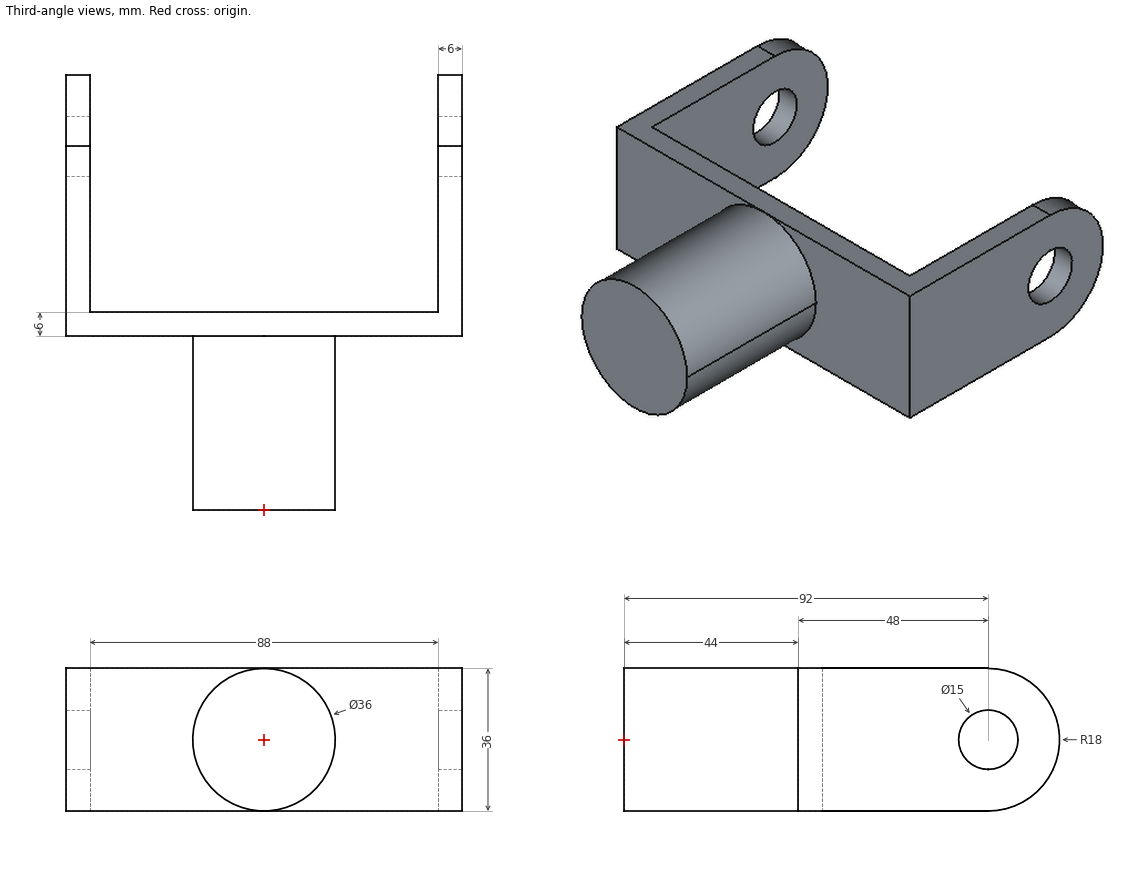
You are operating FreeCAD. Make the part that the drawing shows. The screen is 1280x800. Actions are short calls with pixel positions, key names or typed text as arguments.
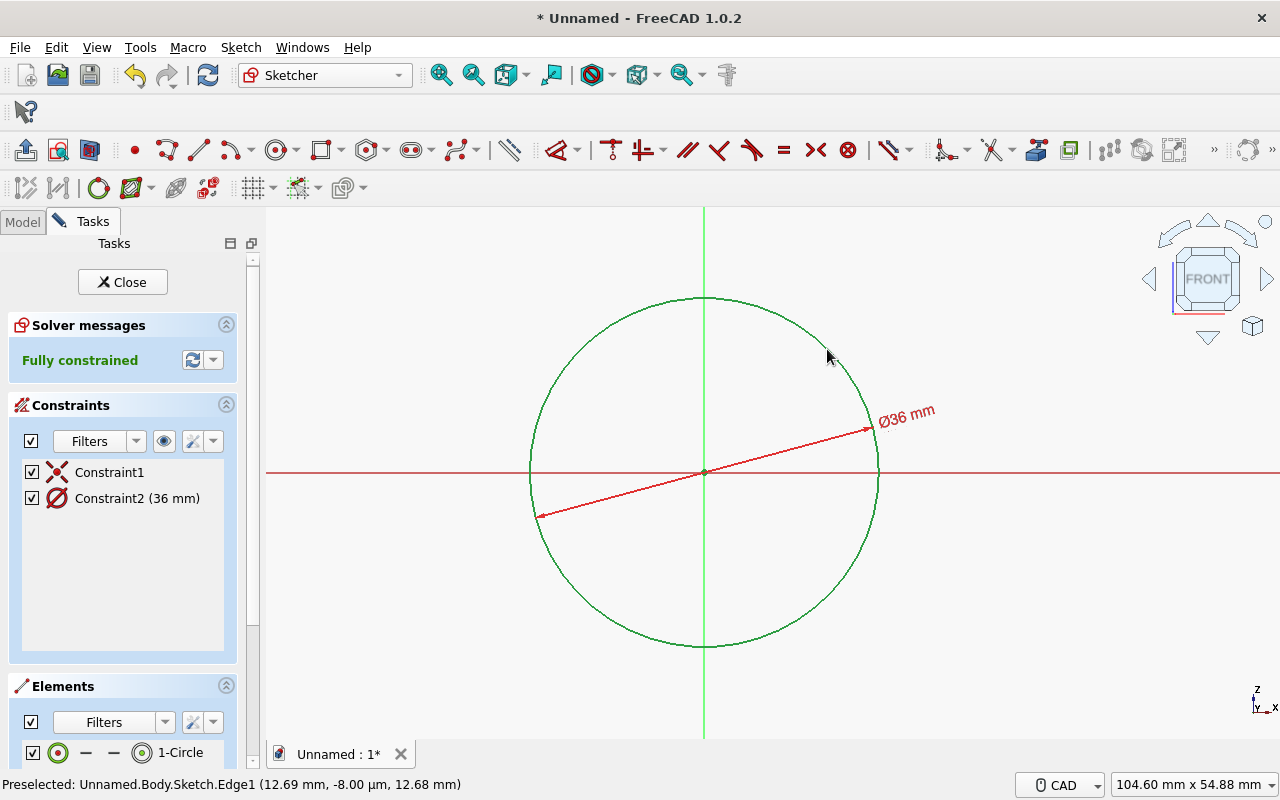
click(123, 282)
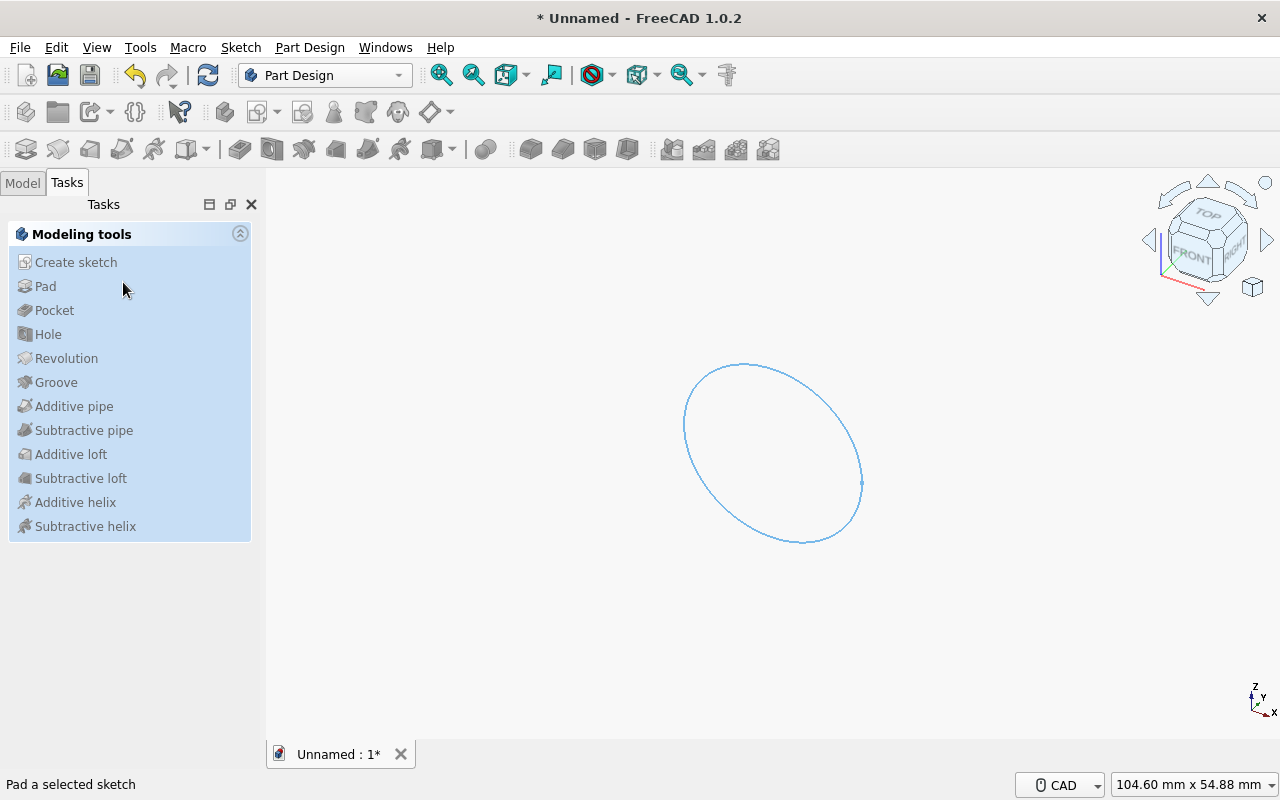
click(26, 150)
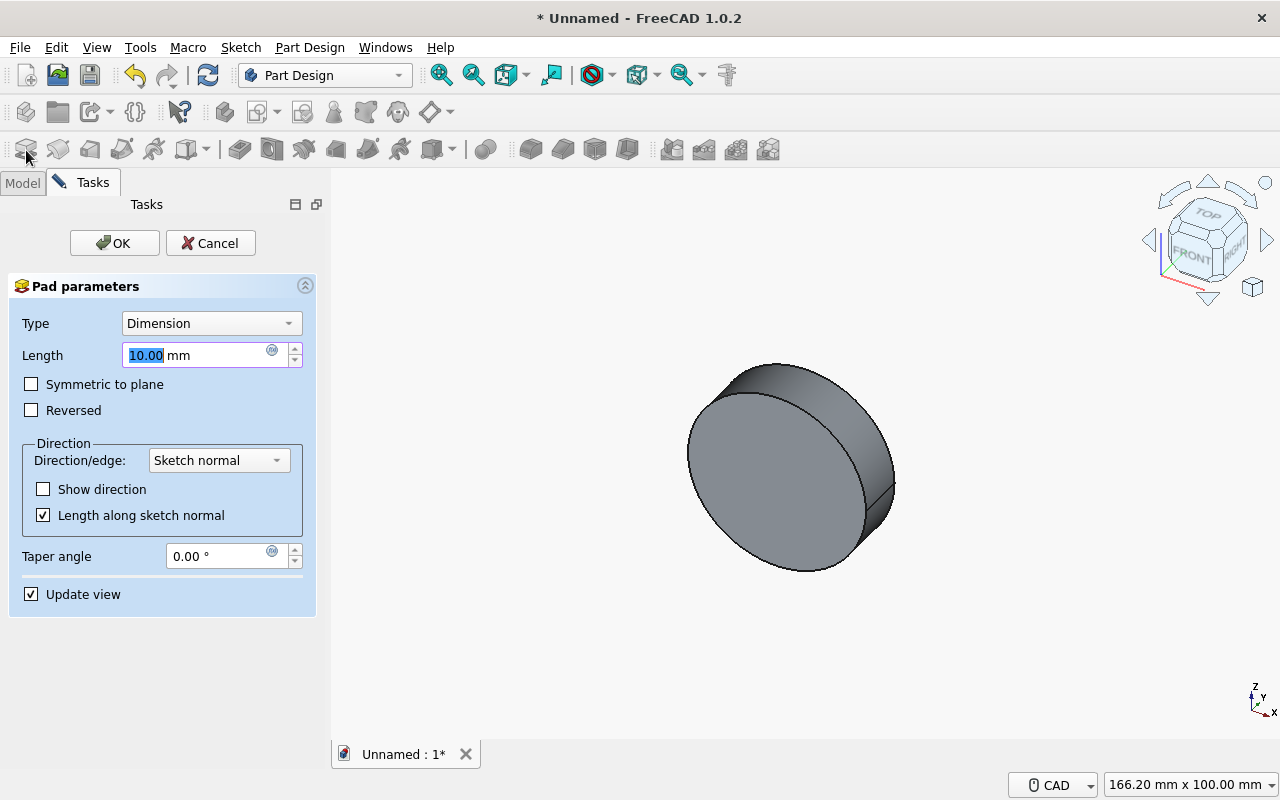
text(44)
key(Tab)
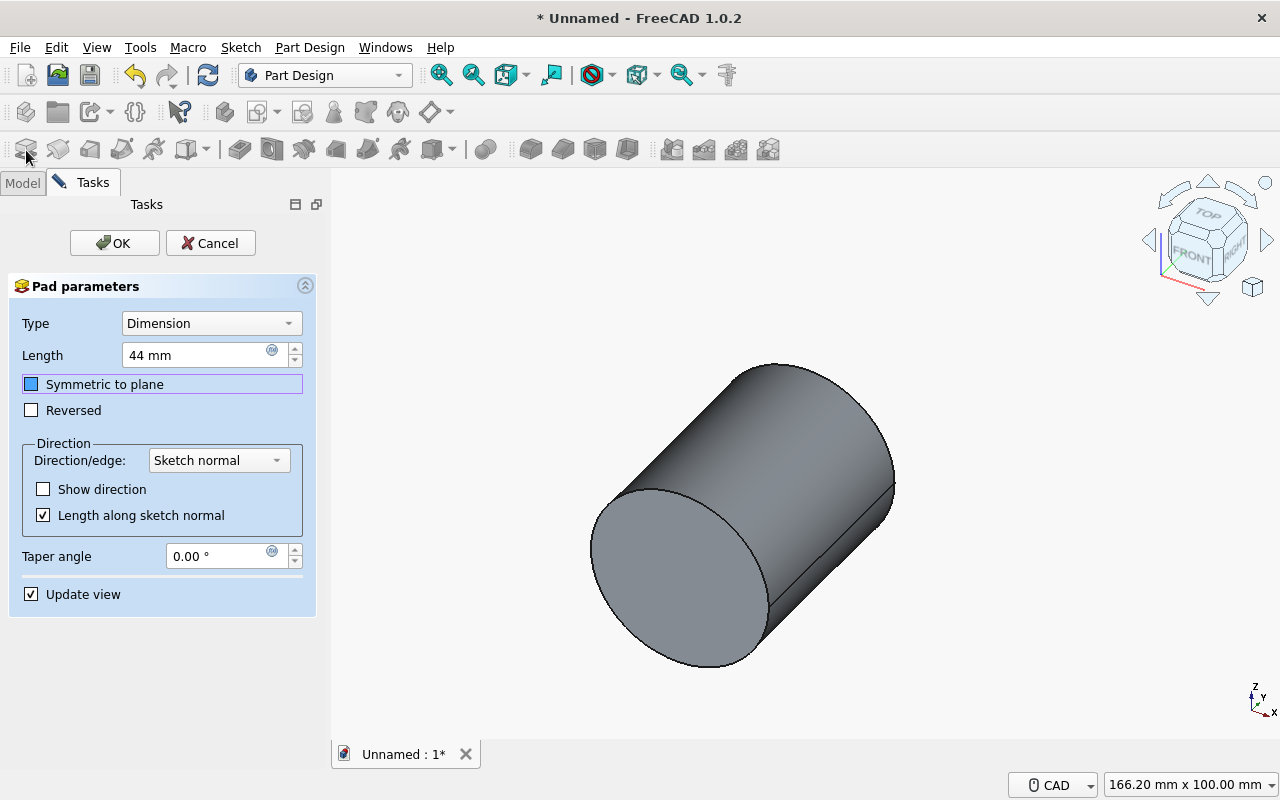
click(30, 410)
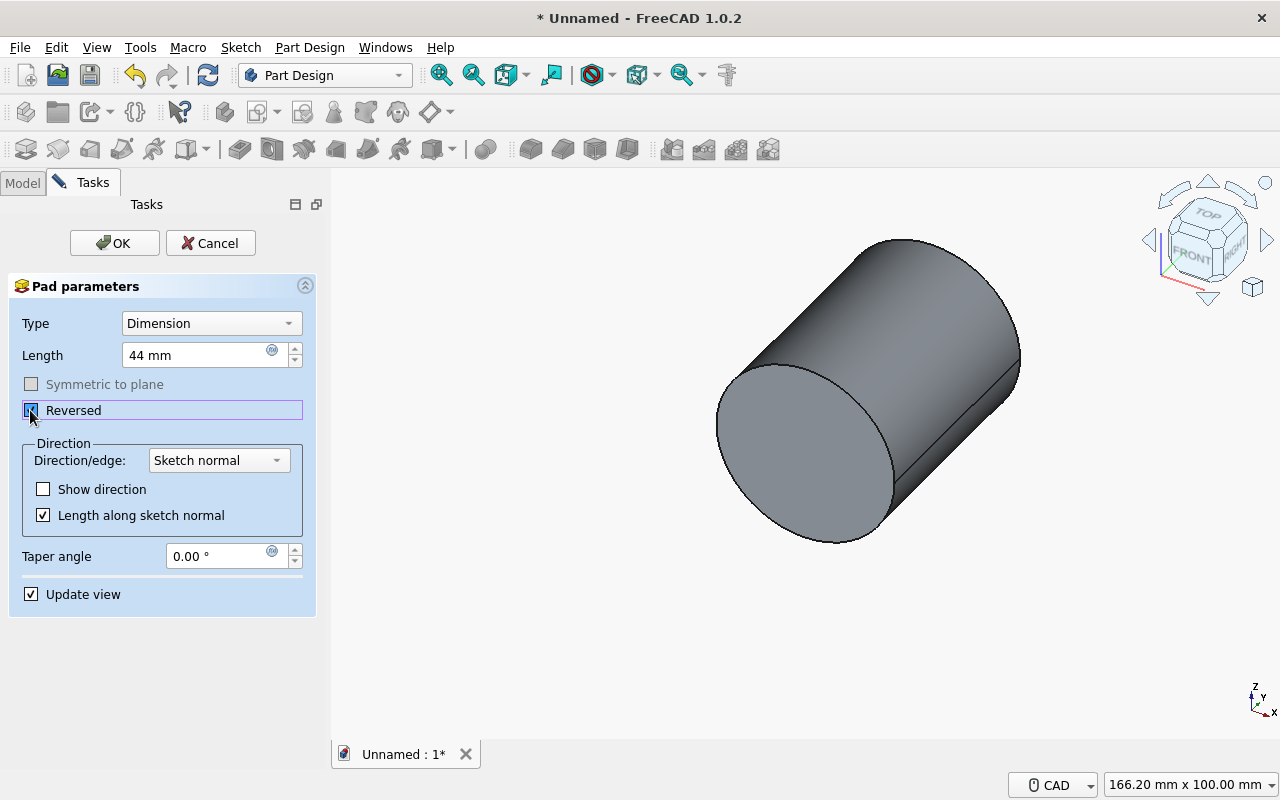
click(115, 243)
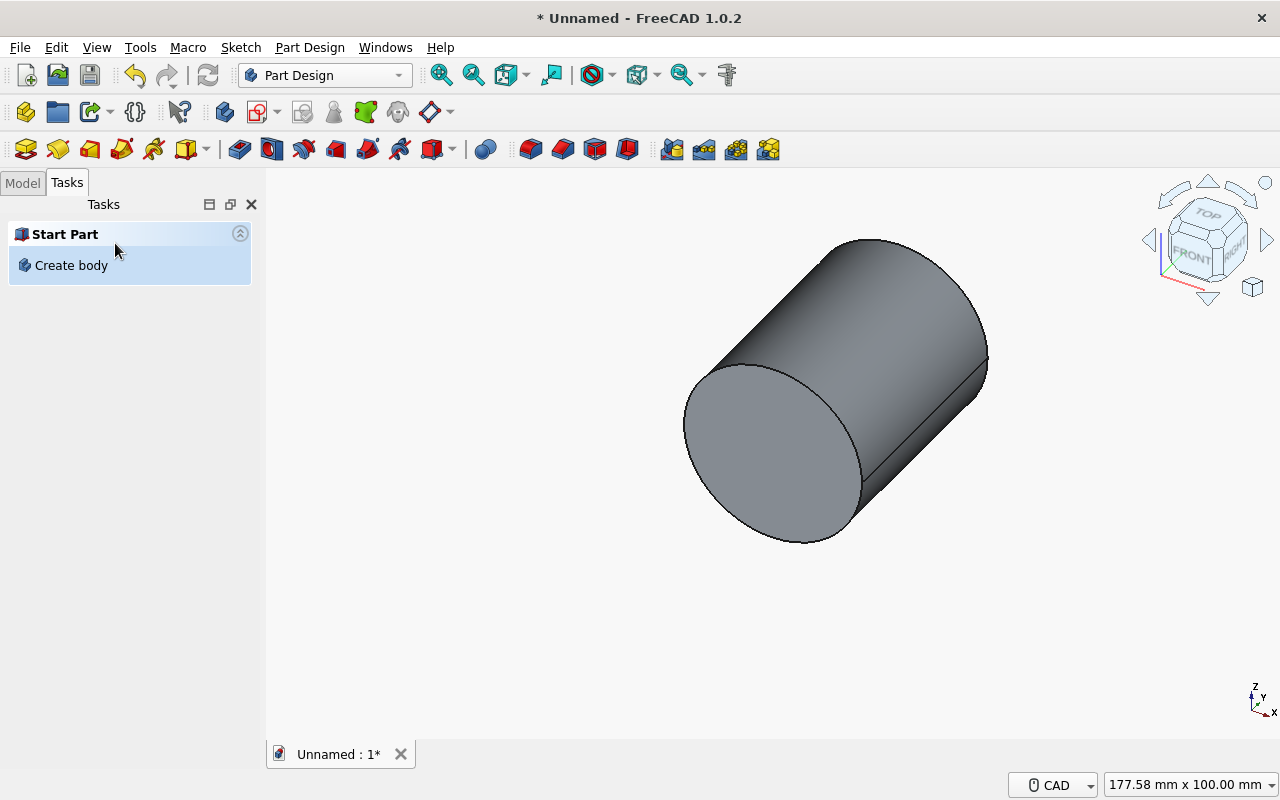
key(4)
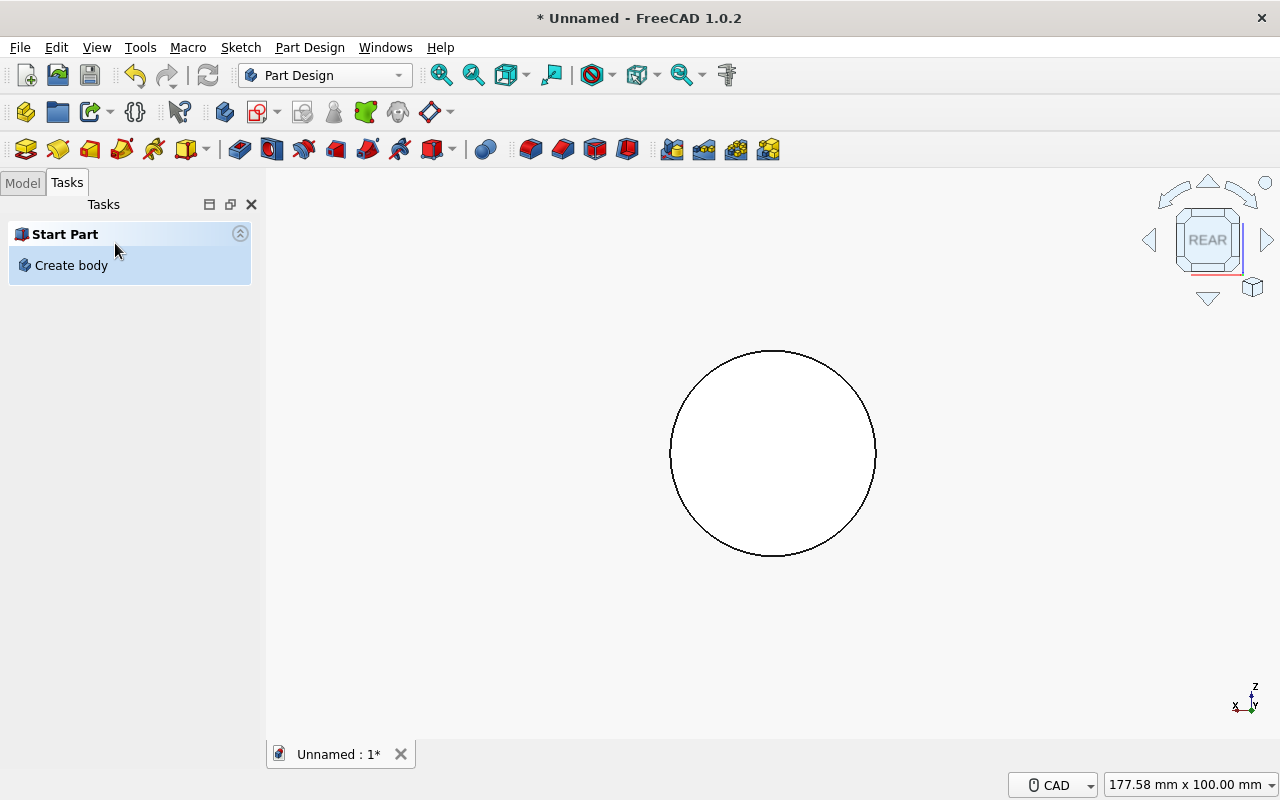
key(v)
key(f)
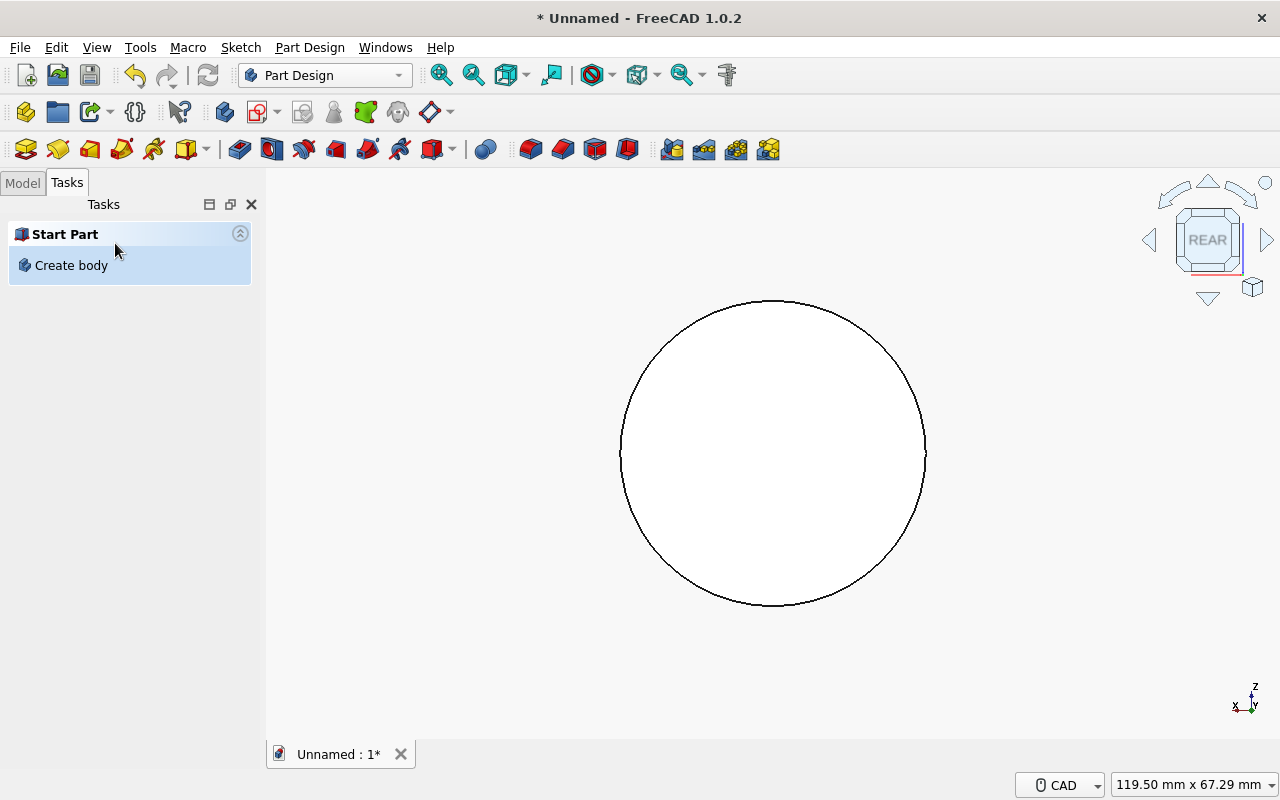
click(773, 453)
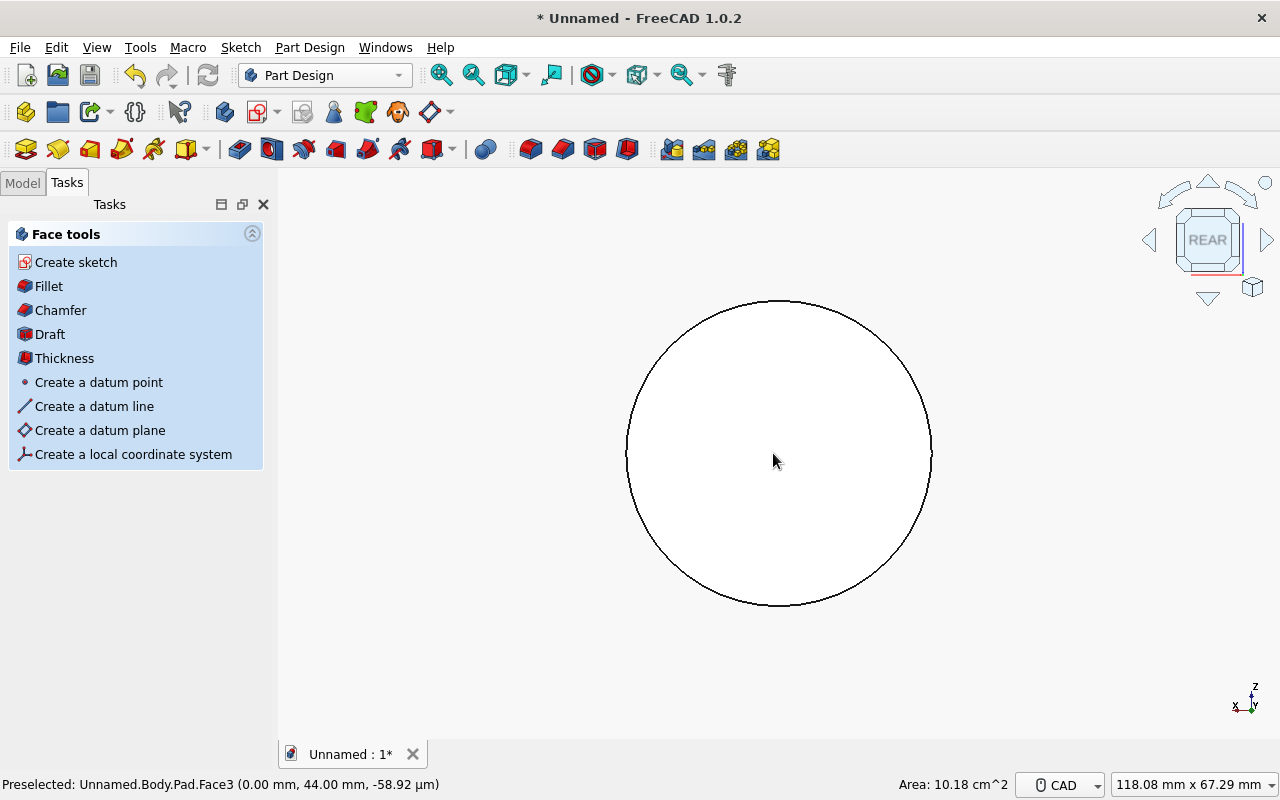
click(258, 112)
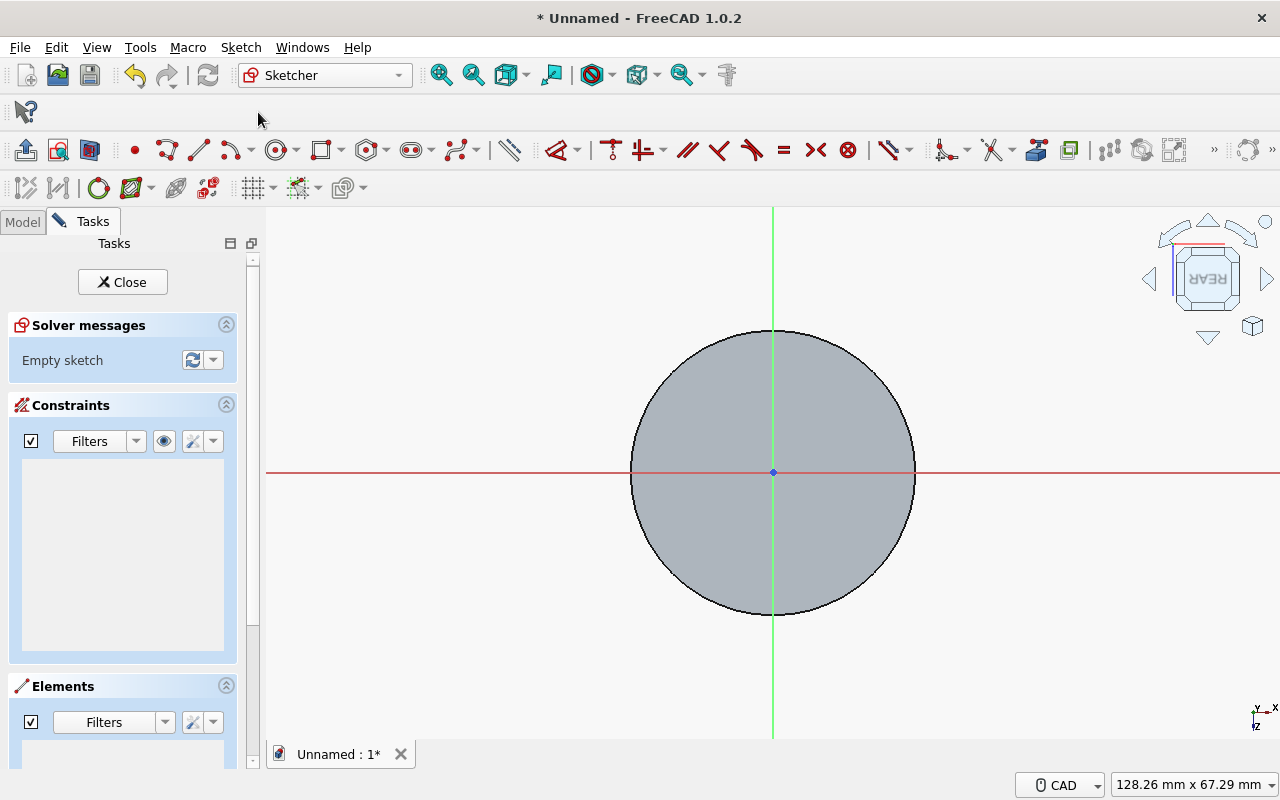
scroll(395, 473, down, 1)